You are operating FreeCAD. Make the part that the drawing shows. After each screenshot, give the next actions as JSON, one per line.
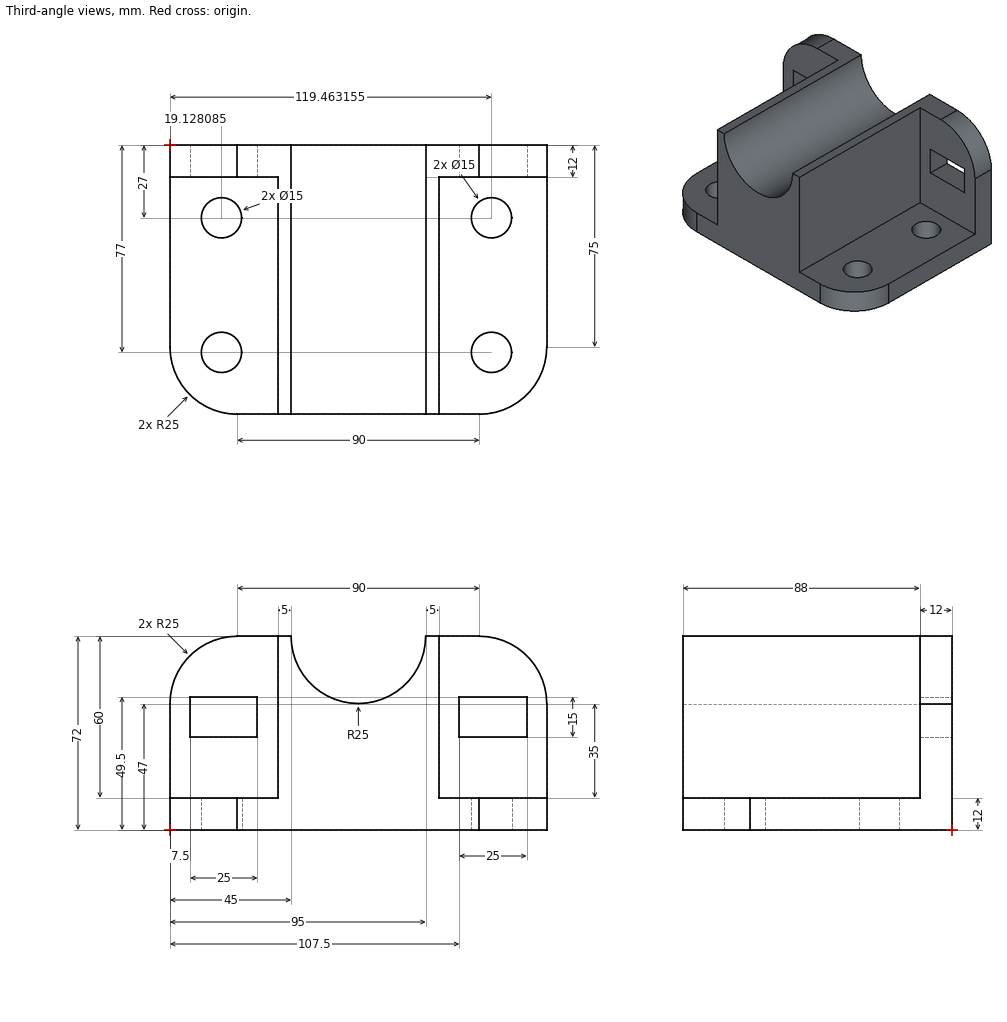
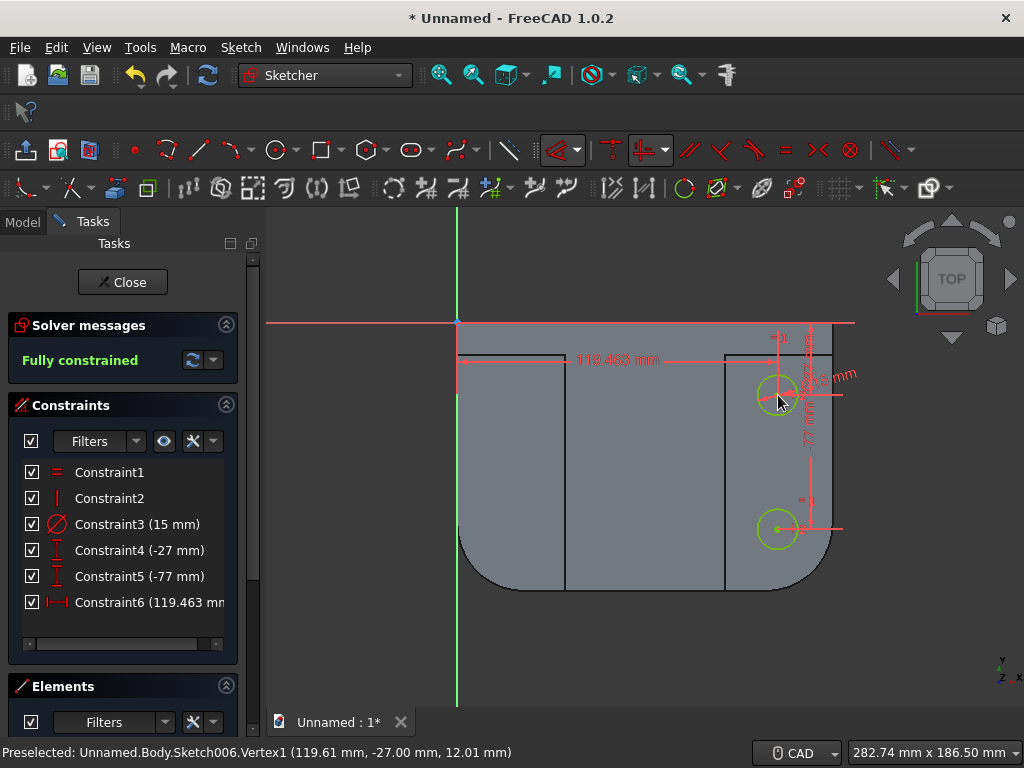
{"action": "left_click", "coordinate": [123, 282]}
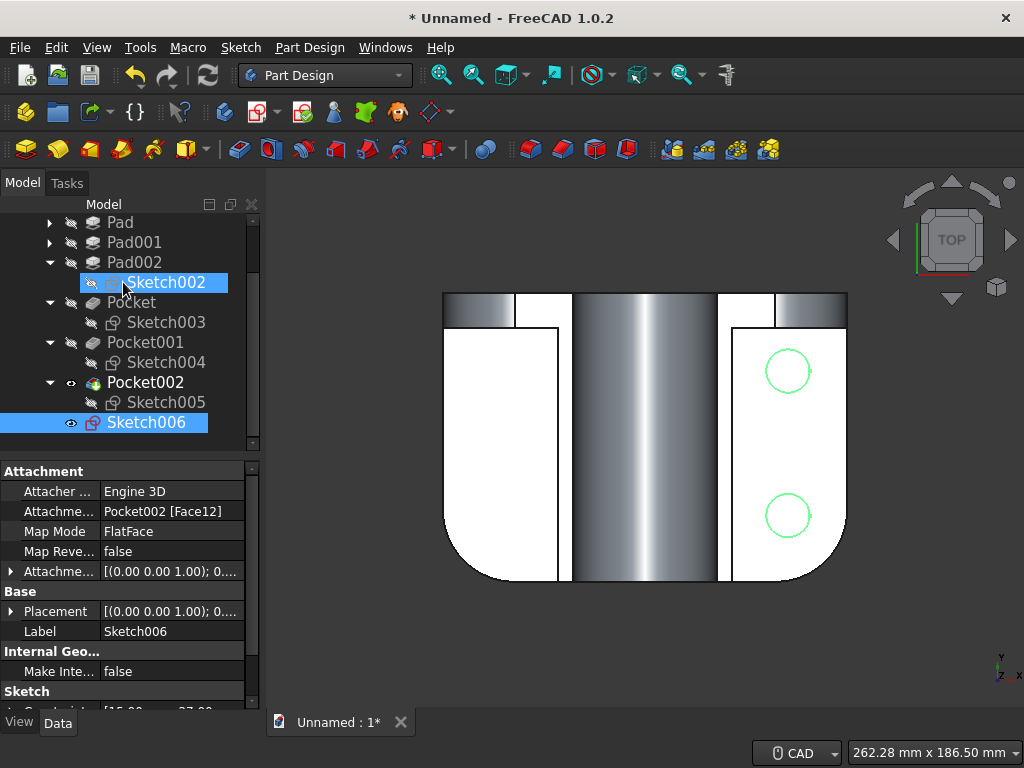
{"action": "left_click", "coordinate": [240, 150]}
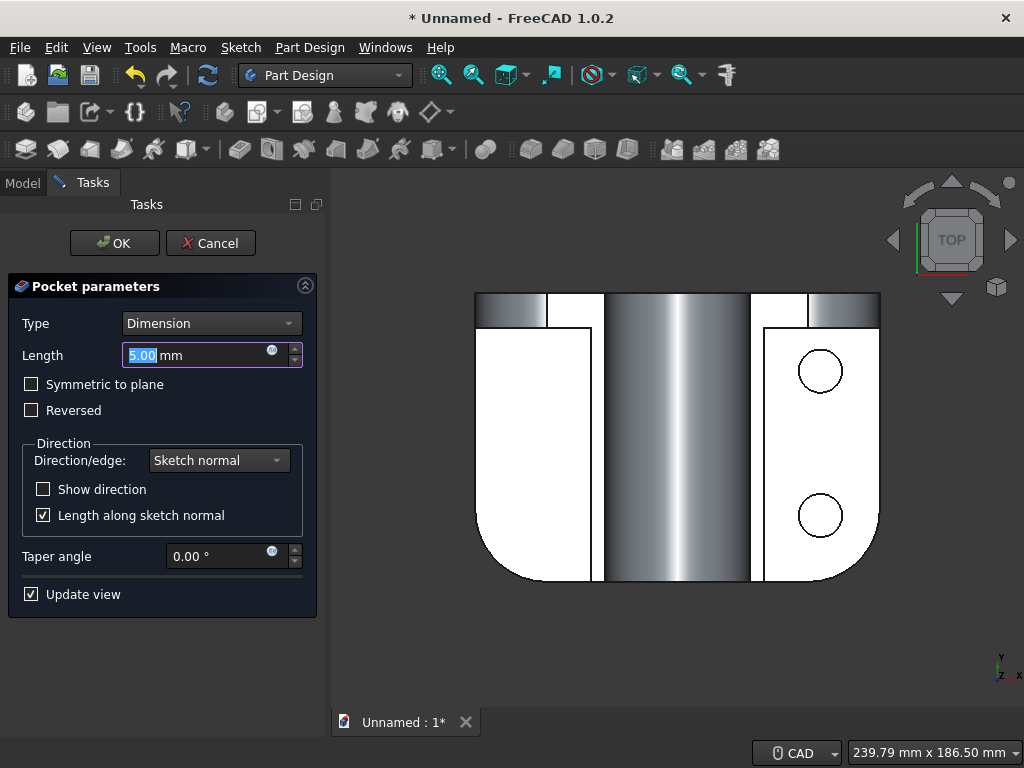
{"action": "type", "text": "12"}
{"action": "key", "text": "Tab"}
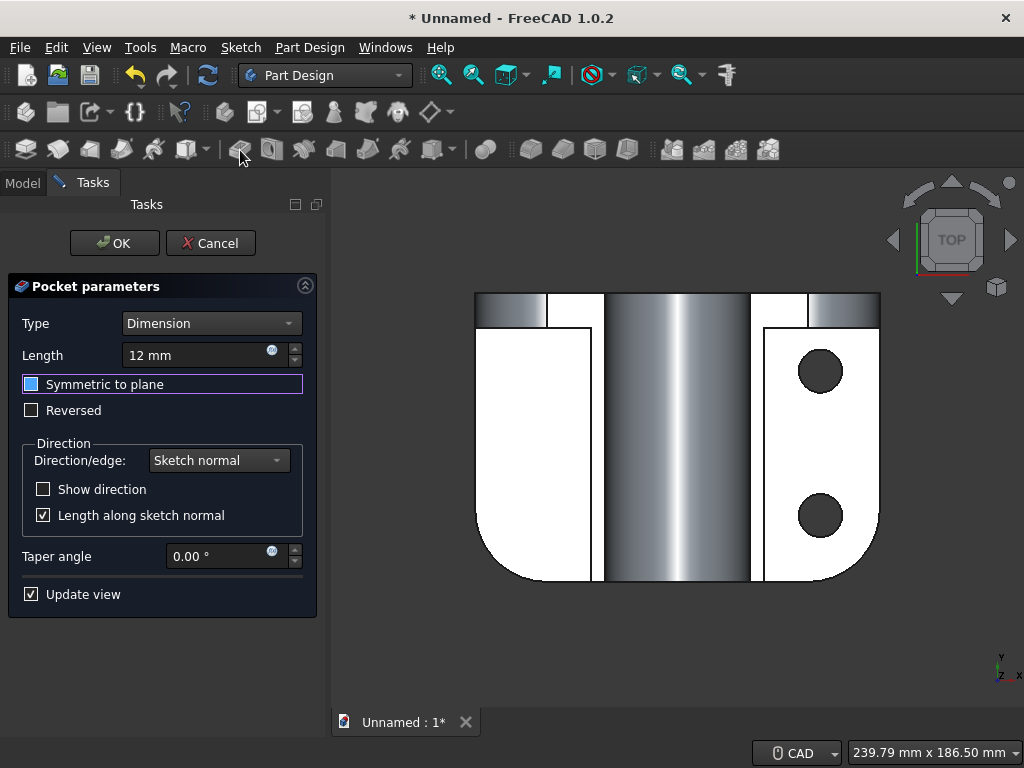
{"action": "left_click", "coordinate": [115, 243]}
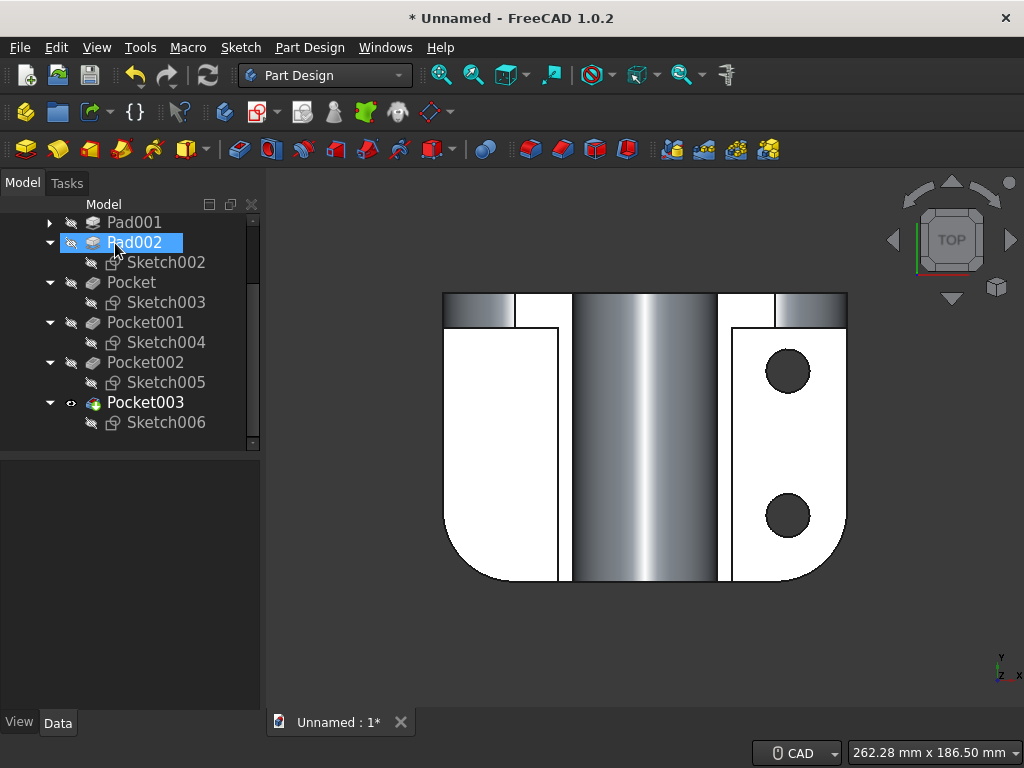
{"action": "left_click", "coordinate": [500, 418]}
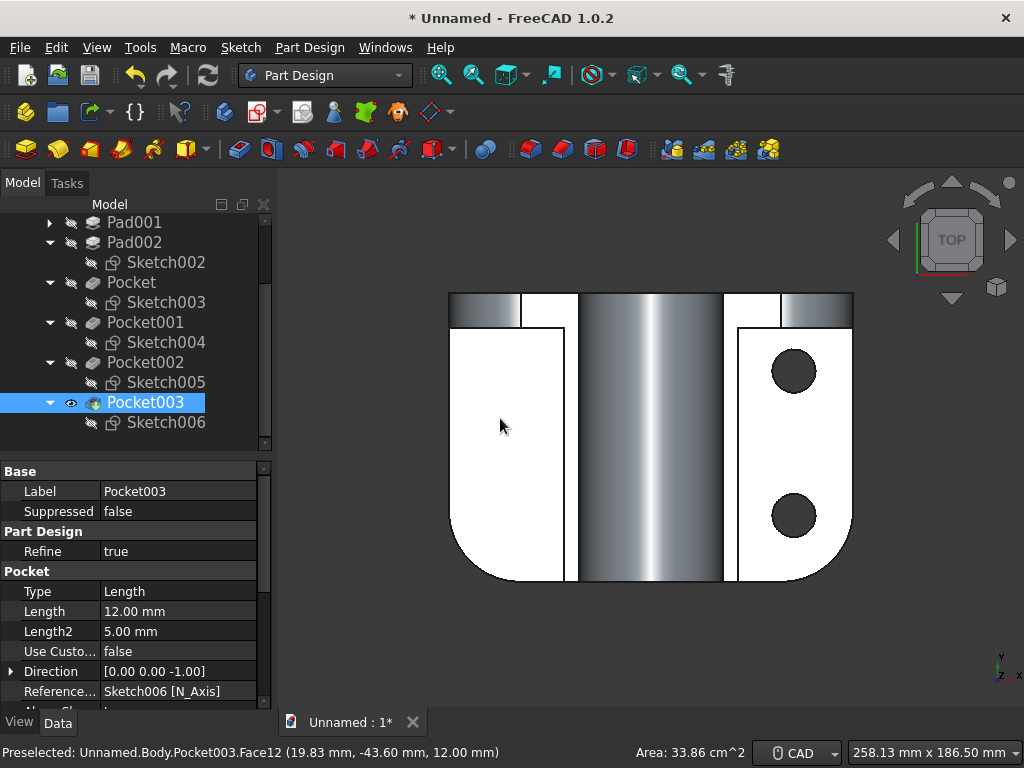
{"action": "left_click", "coordinate": [258, 112]}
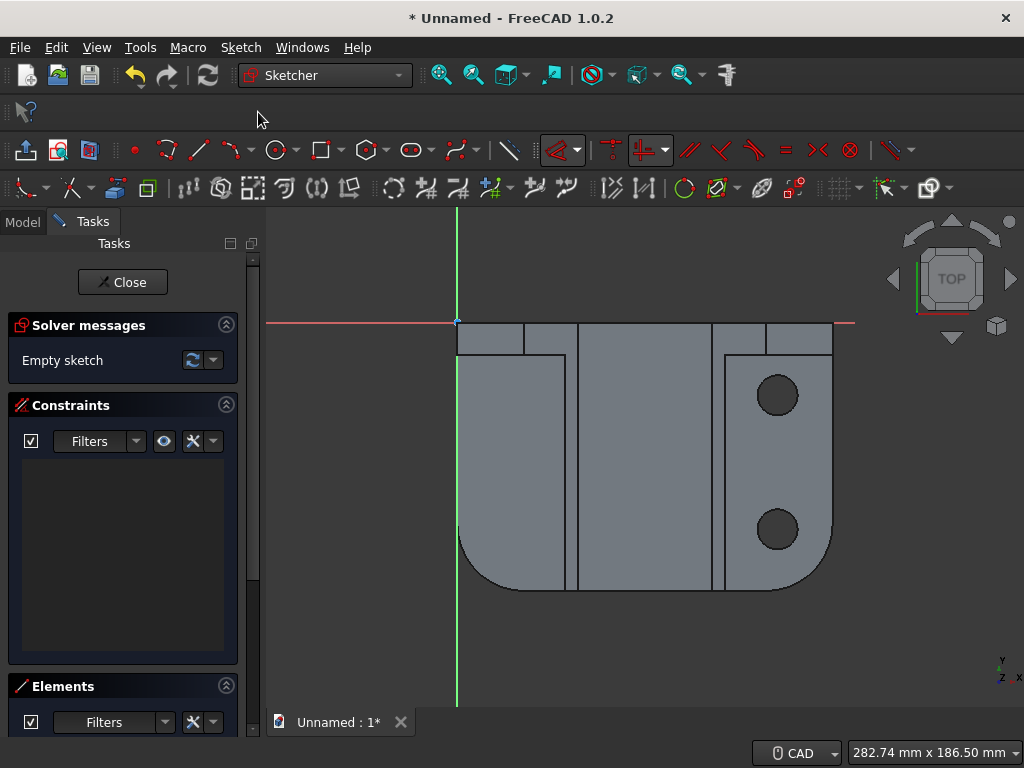
{"action": "key", "text": "q s"}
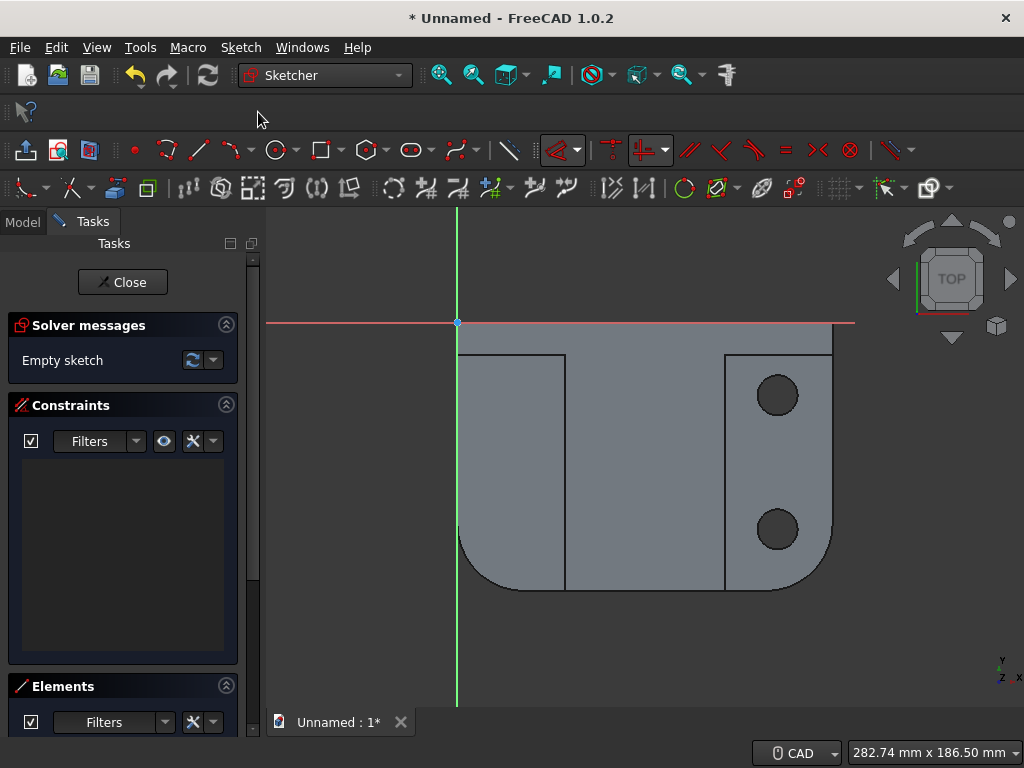
{"action": "scroll", "coordinate": [323, 394], "scroll_direction": "up", "scroll_amount": 2}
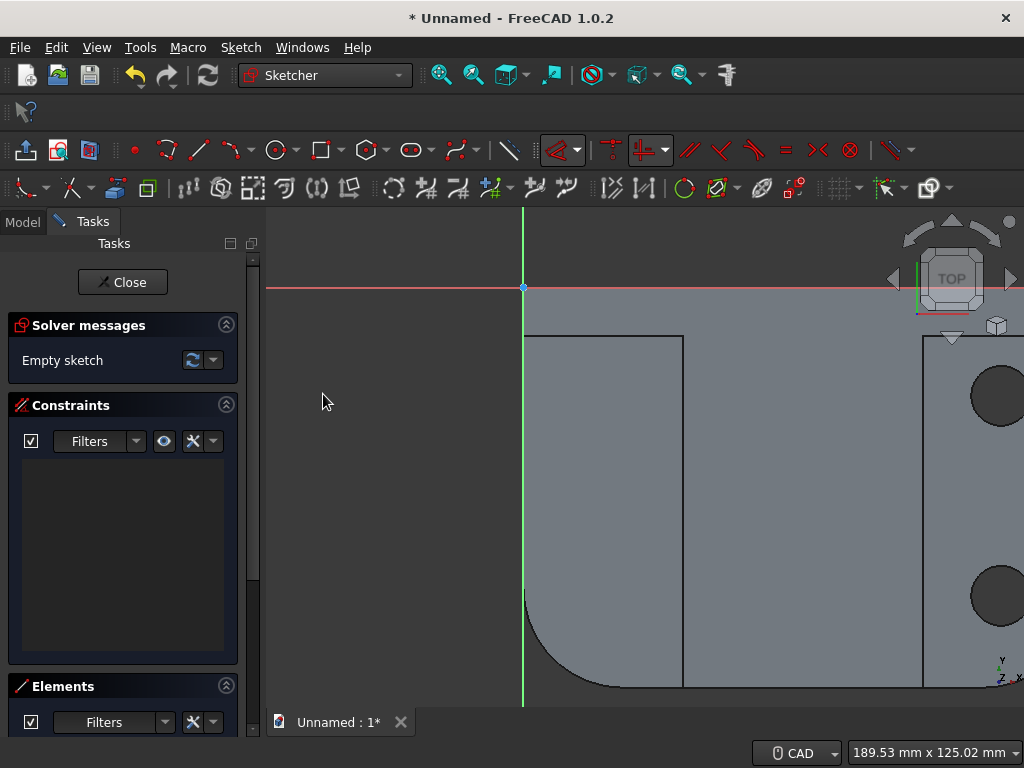
{"action": "left_click", "coordinate": [276, 150]}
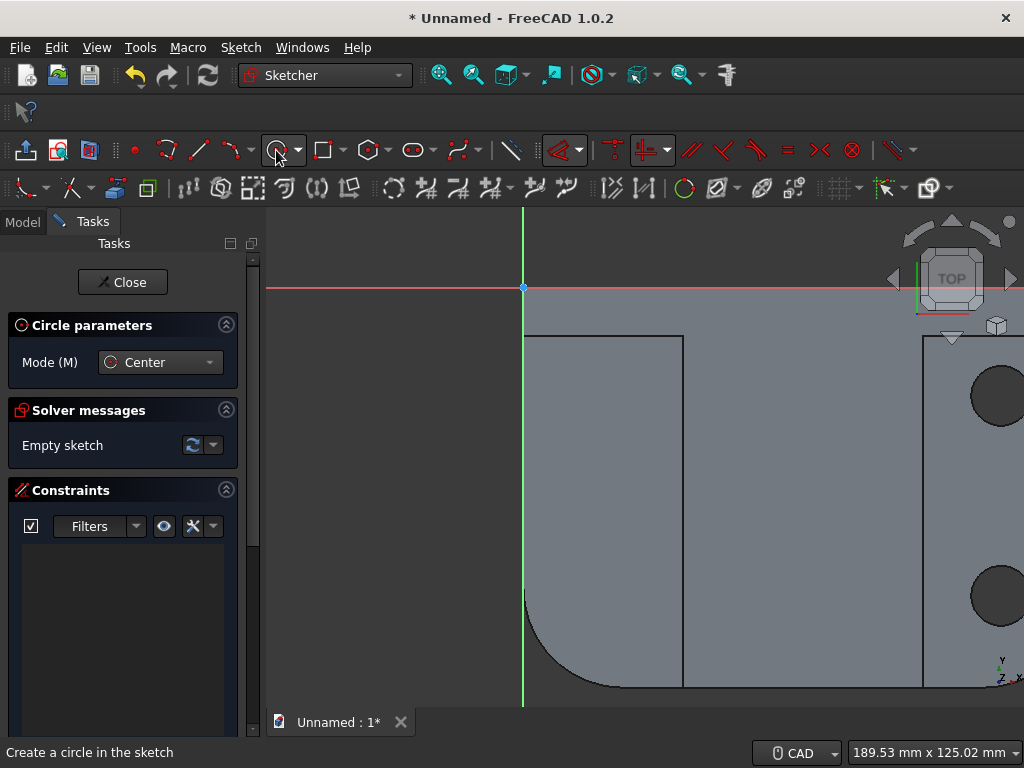
{"action": "left_click", "coordinate": [600, 396]}
{"action": "left_click", "coordinate": [621, 375]}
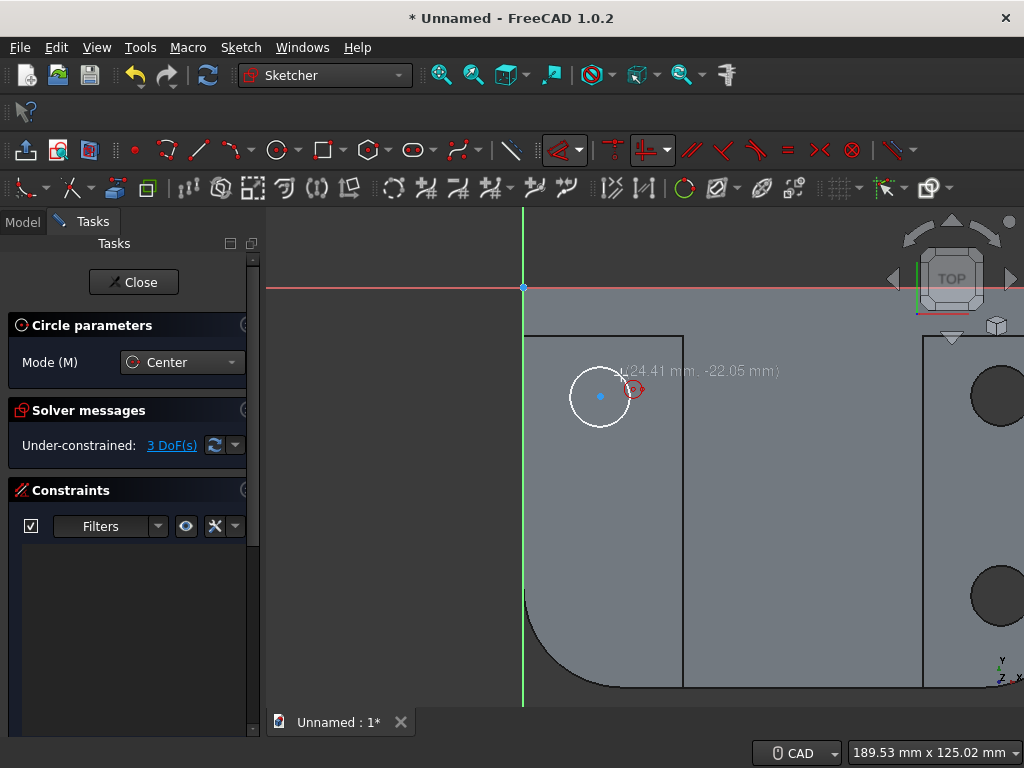
{"action": "left_click", "coordinate": [600, 596]}
{"action": "left_click", "coordinate": [621, 575]}
{"action": "key", "text": "Escape"}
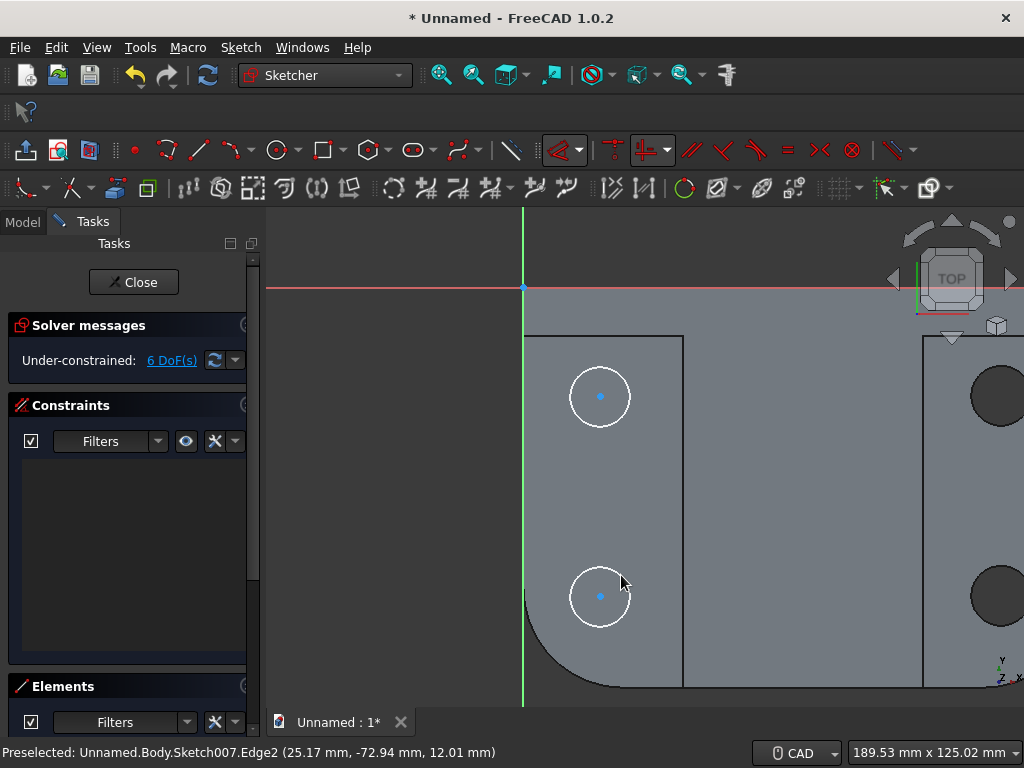
{"action": "left_click", "coordinate": [621, 376]}